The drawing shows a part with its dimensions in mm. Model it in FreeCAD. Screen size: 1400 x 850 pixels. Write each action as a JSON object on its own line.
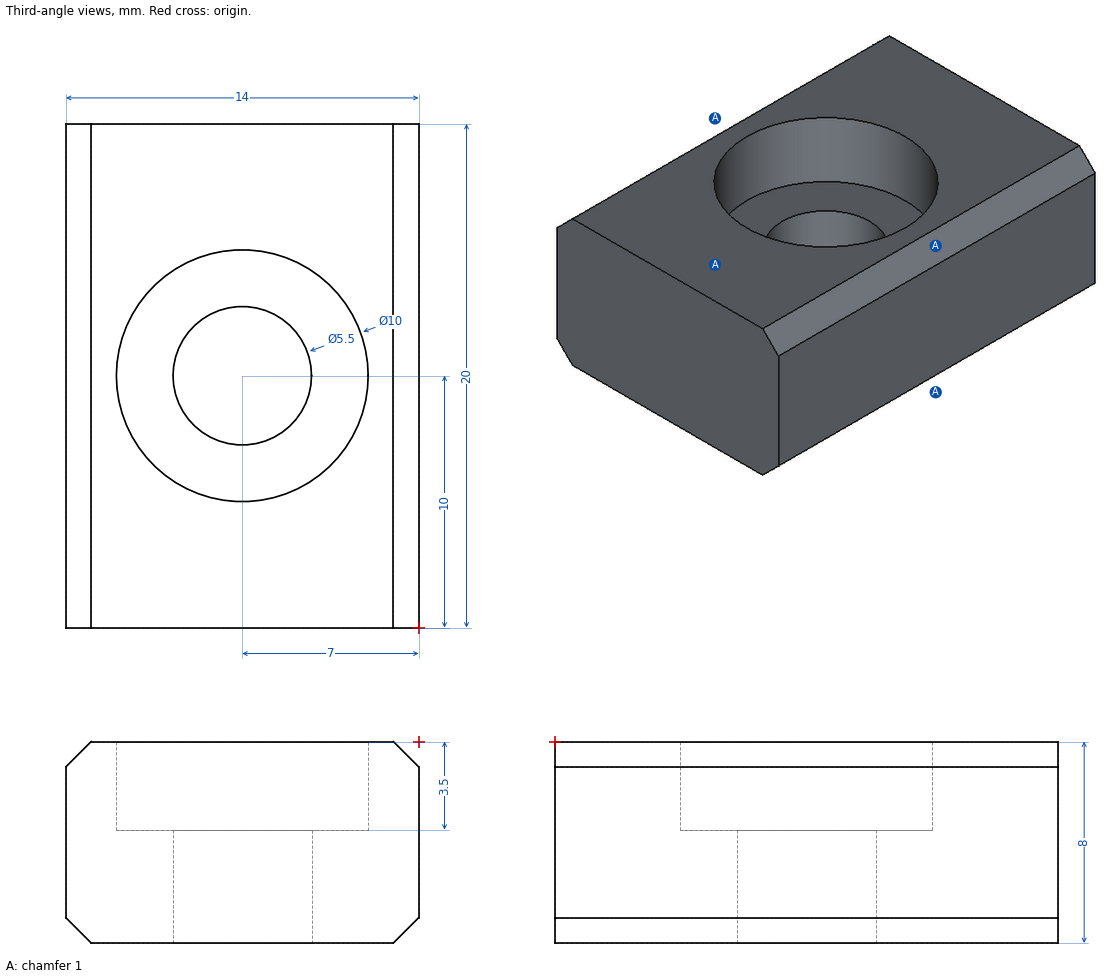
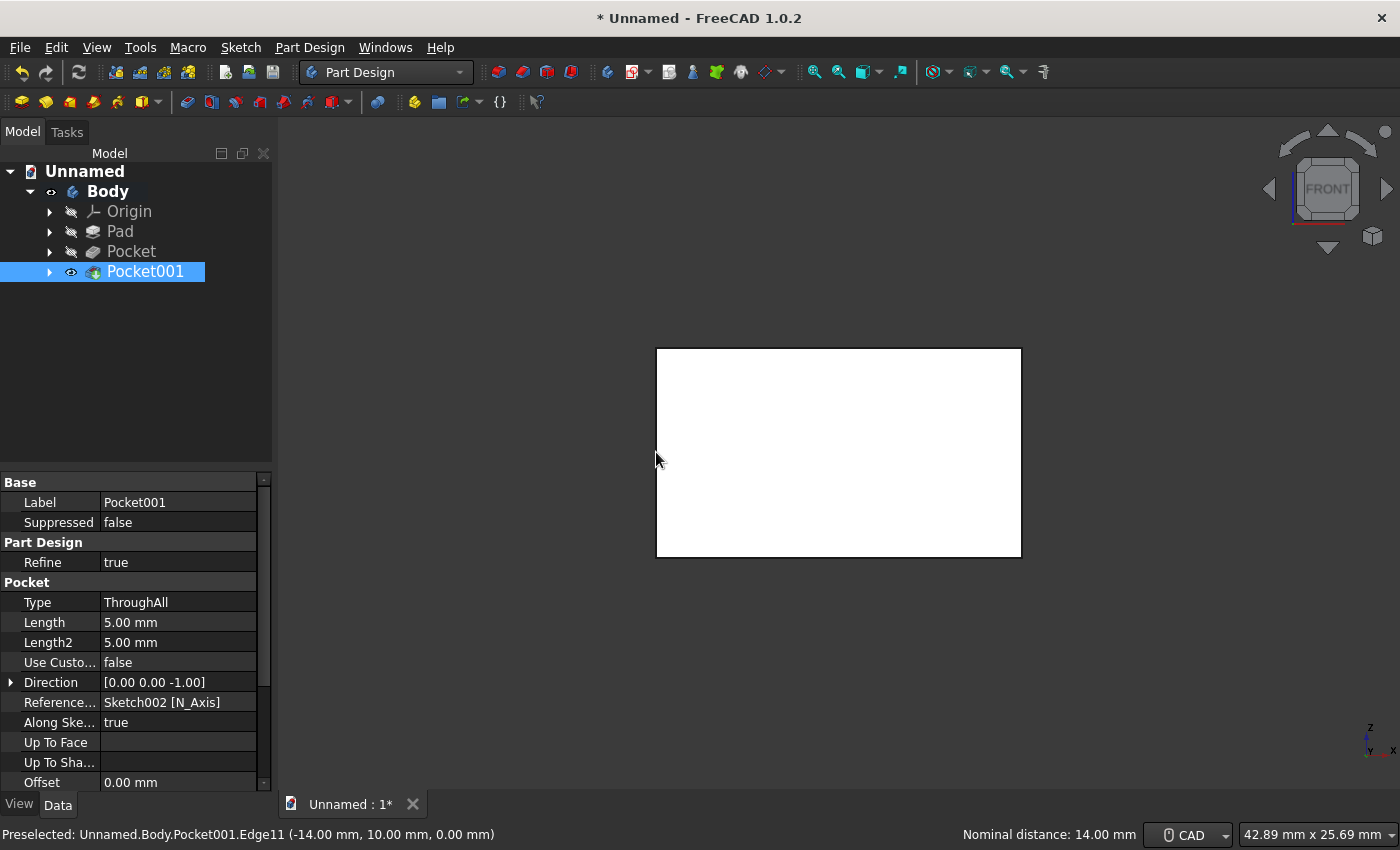
{"action": "key", "text": "v f"}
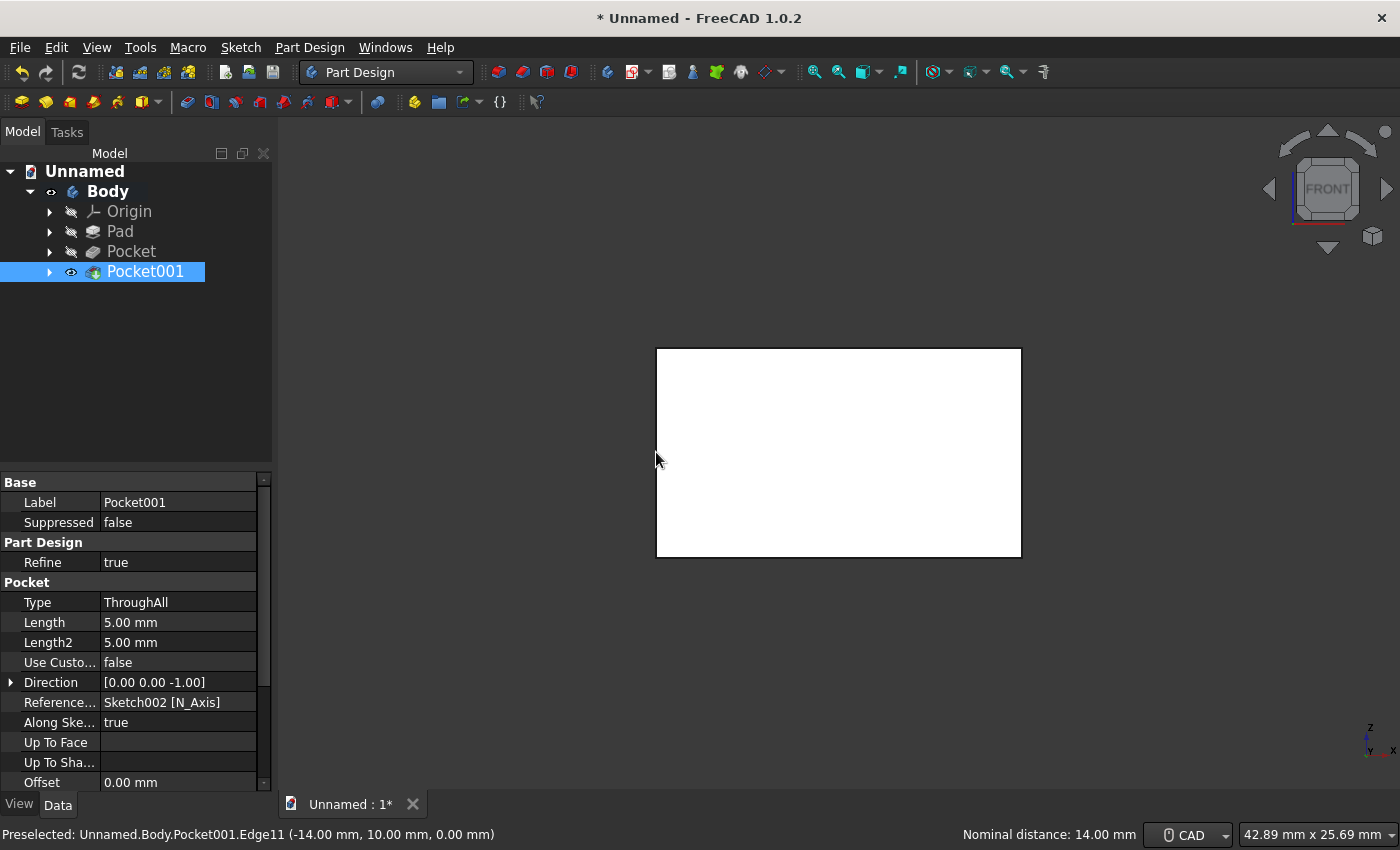
{"action": "key", "text": "3"}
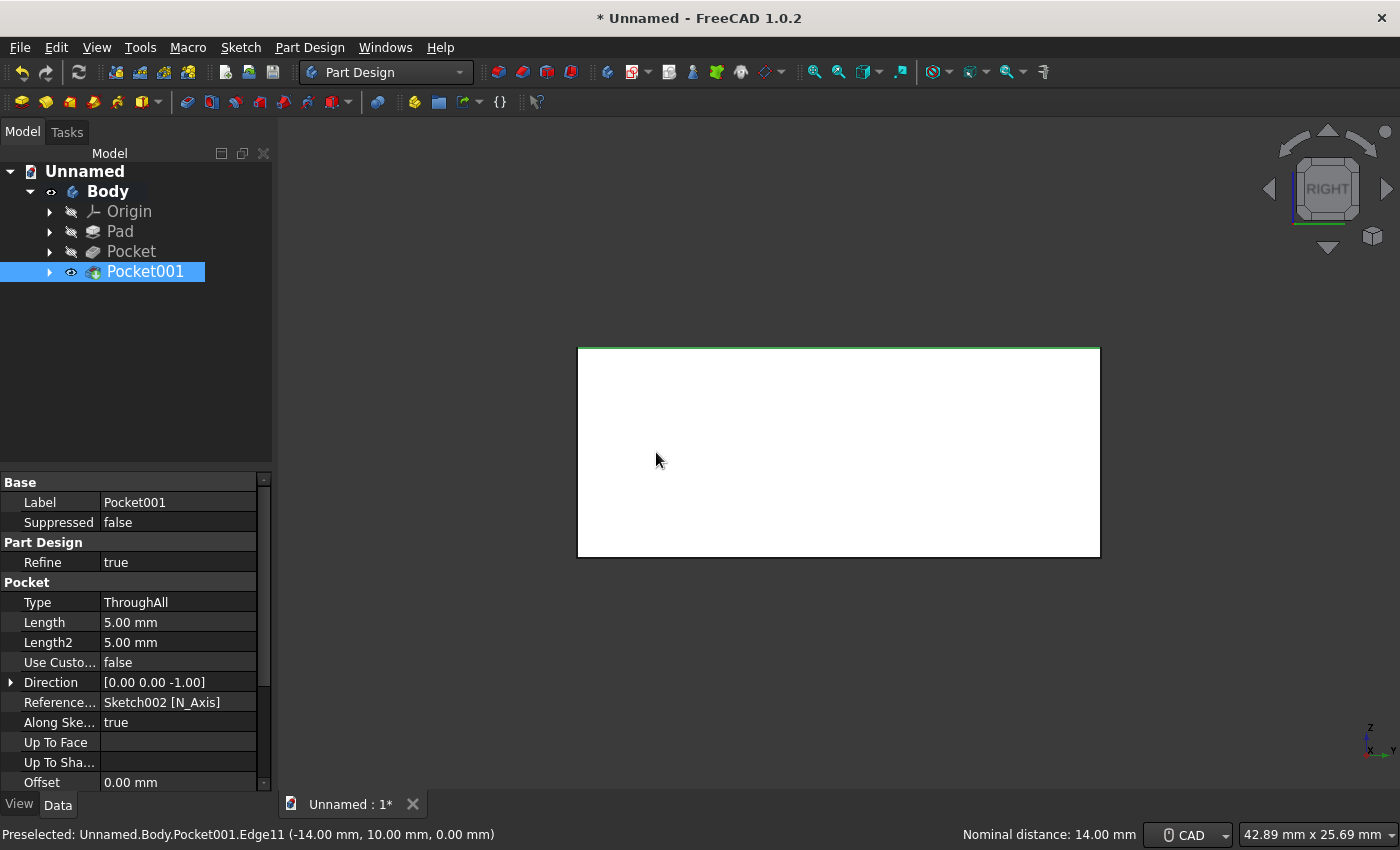
{"action": "left_click", "coordinate": [839, 557], "text": "ctrl"}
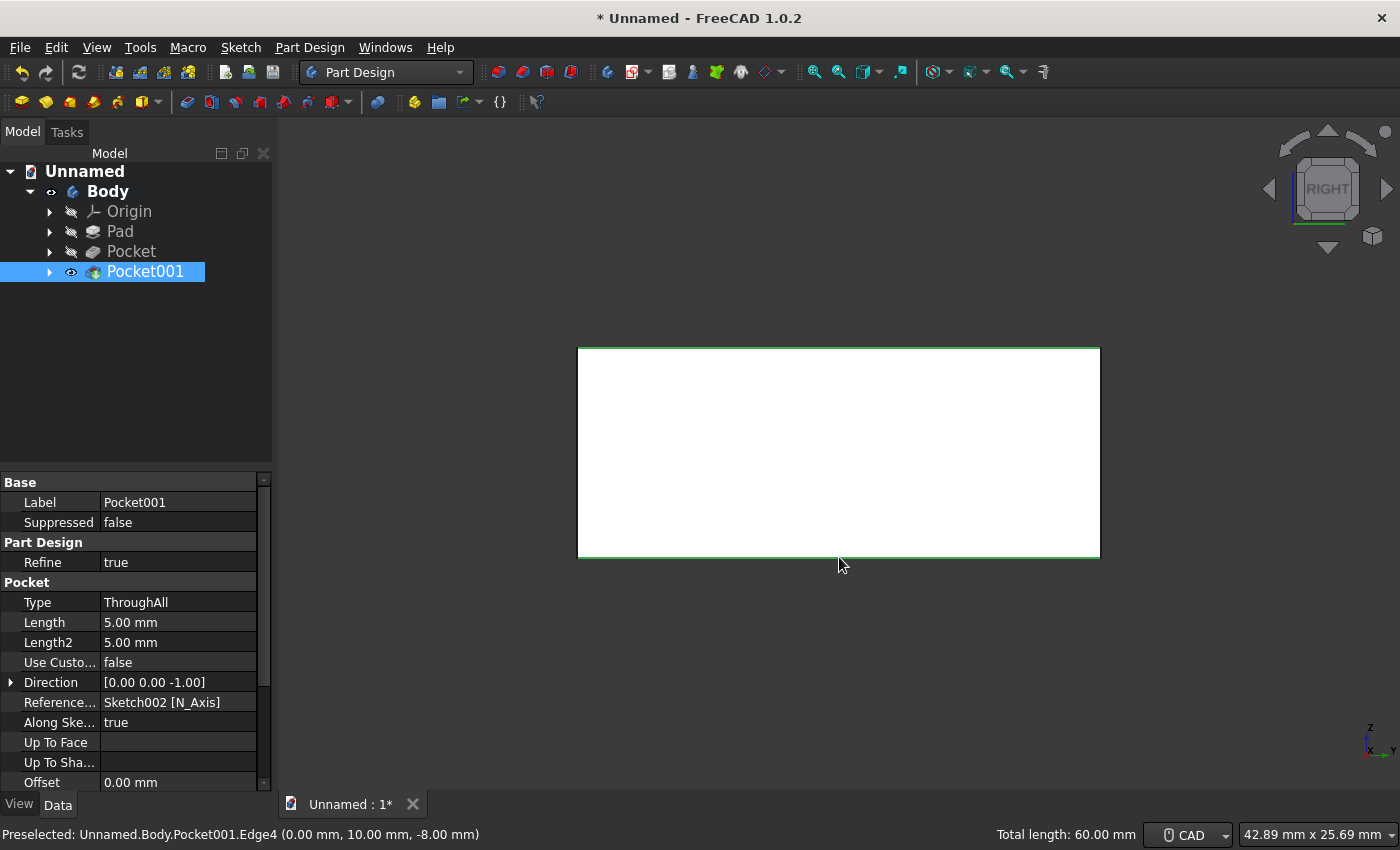
{"action": "key", "text": "5"}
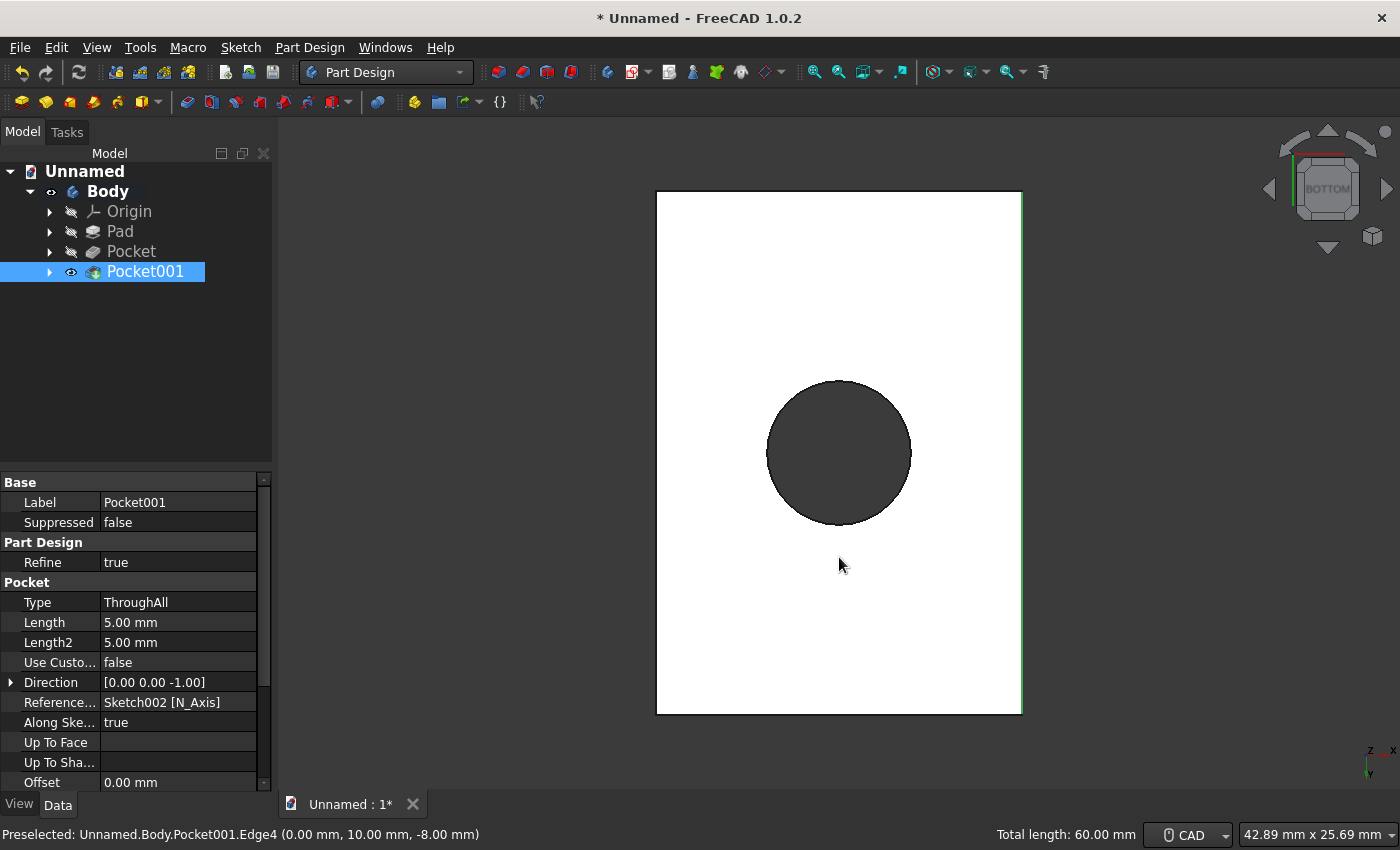
{"action": "left_click", "coordinate": [656, 452], "text": "ctrl"}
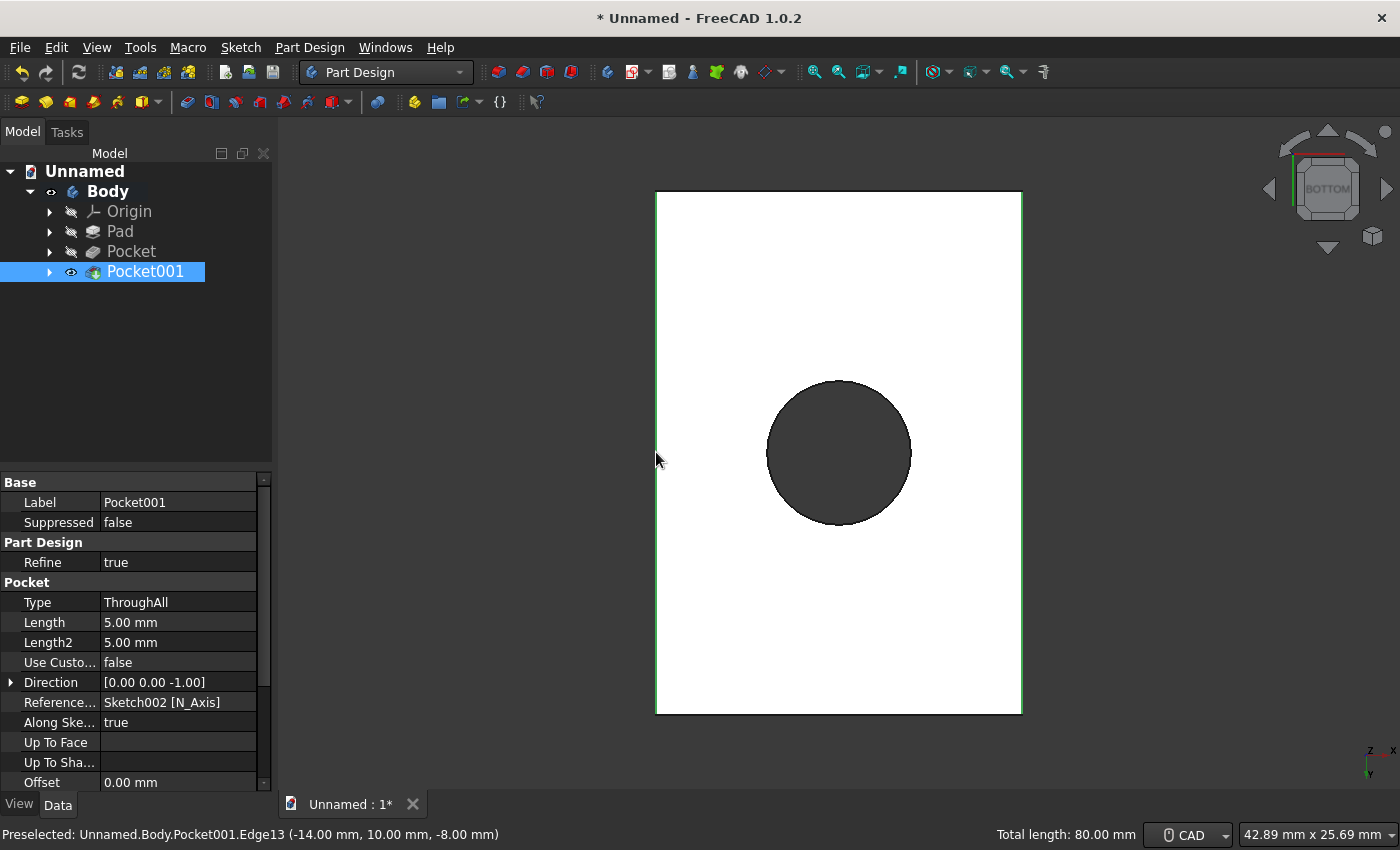
{"action": "left_click", "coordinate": [524, 72]}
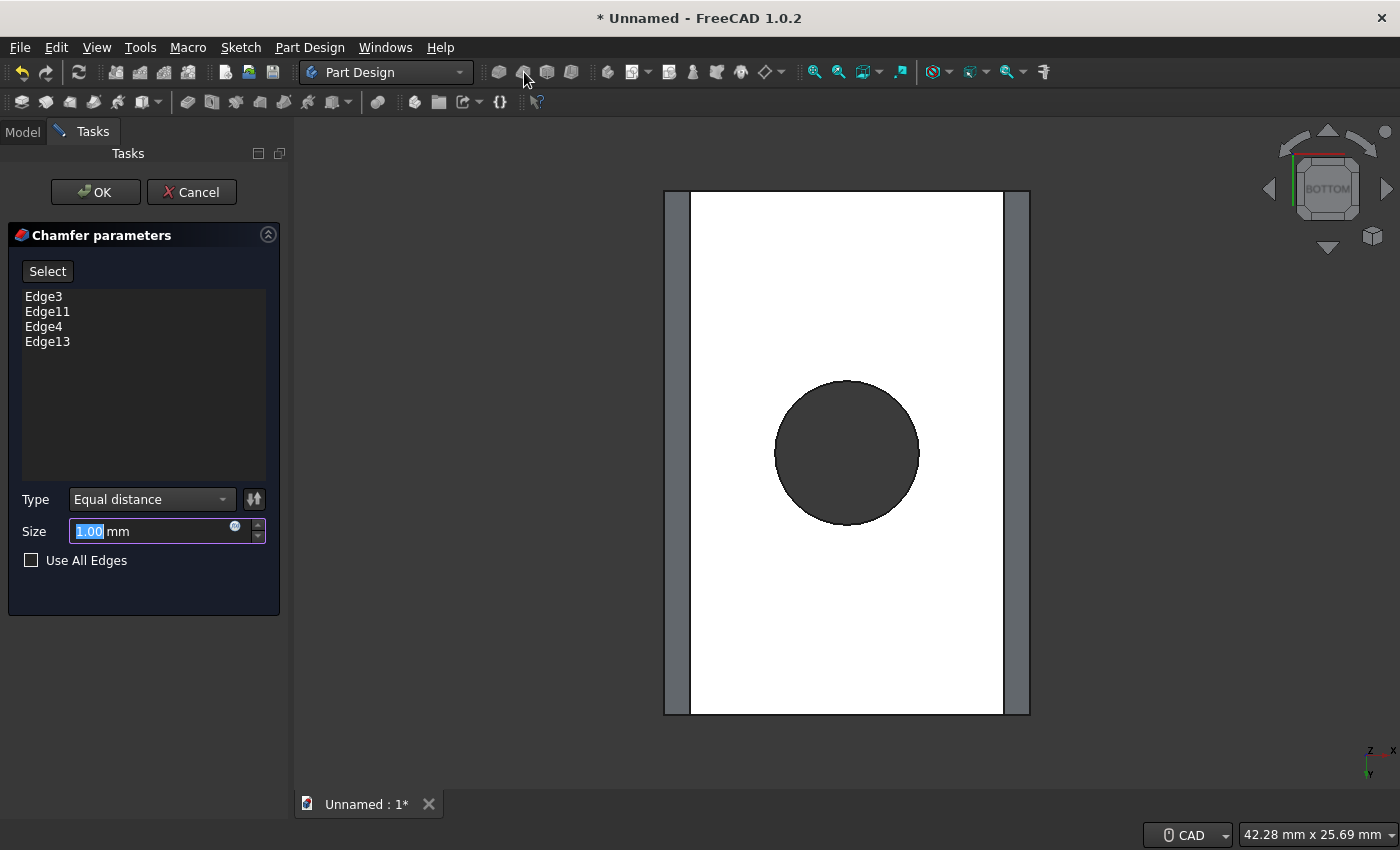
{"action": "type", "text": "1"}
{"action": "key", "text": "Tab"}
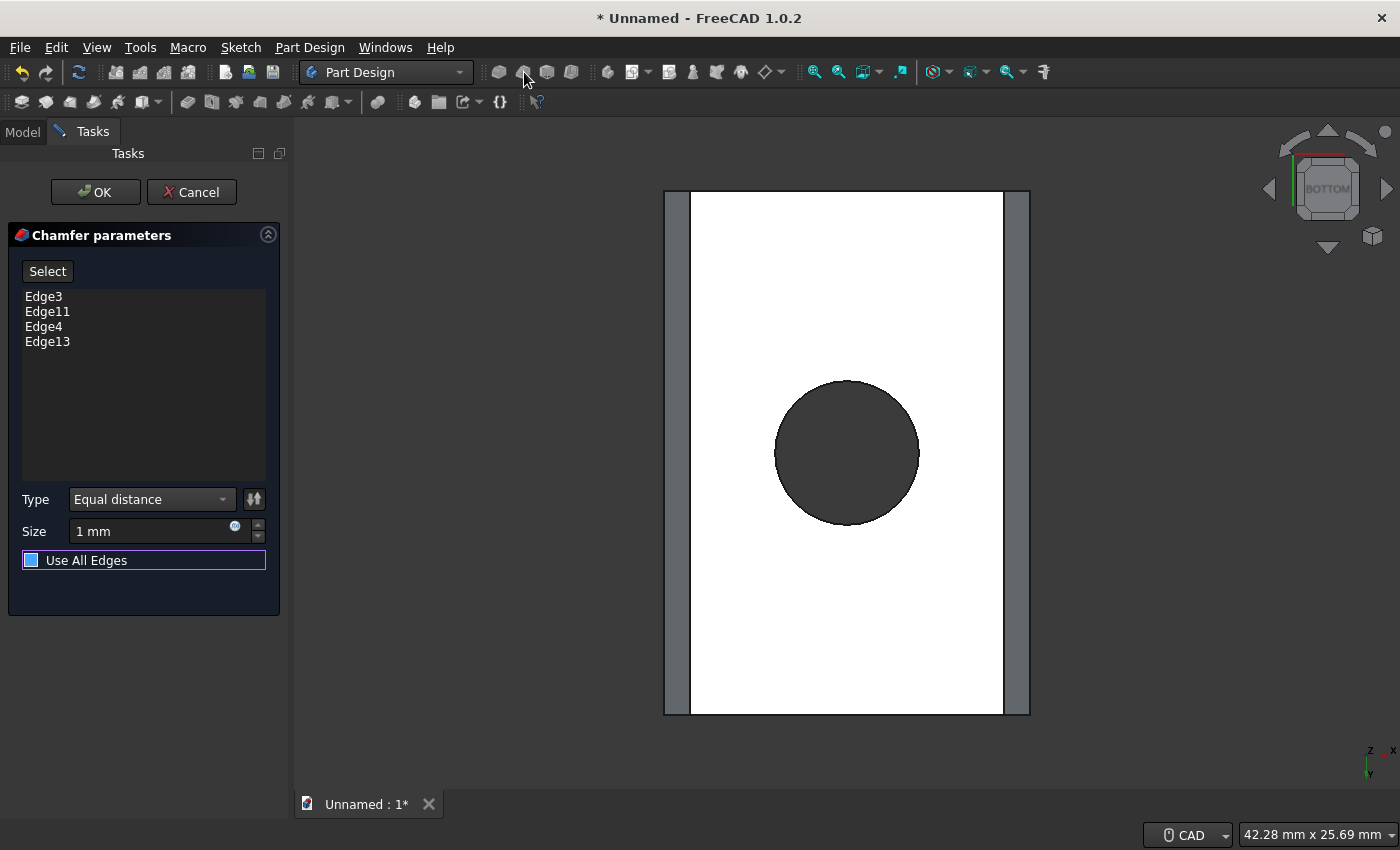
{"action": "left_click", "coordinate": [96, 192]}